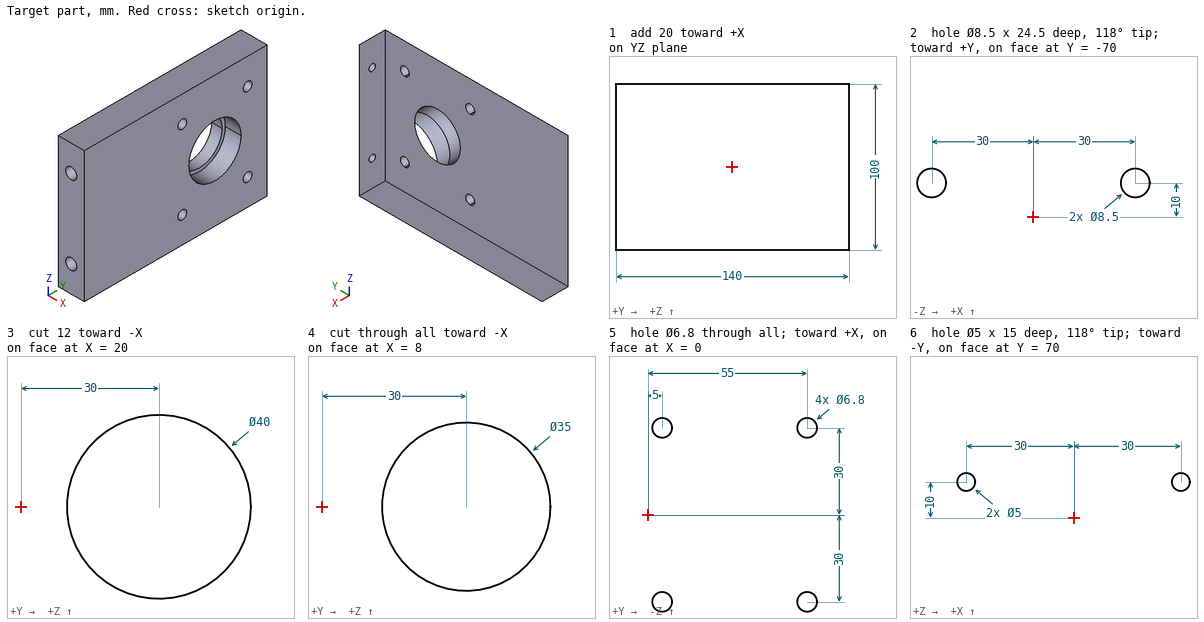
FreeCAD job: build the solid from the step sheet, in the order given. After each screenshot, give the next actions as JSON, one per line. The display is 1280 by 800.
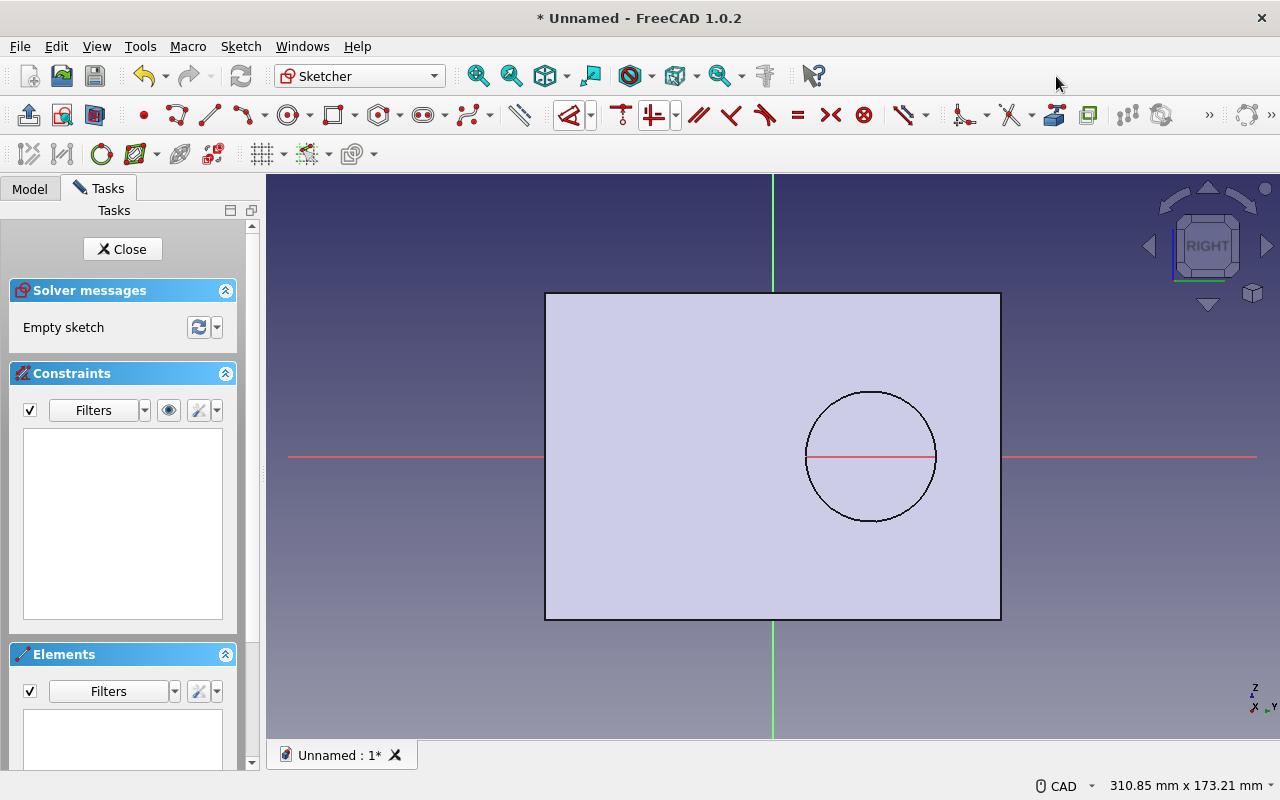
{"action": "left_click", "coordinate": [95, 116]}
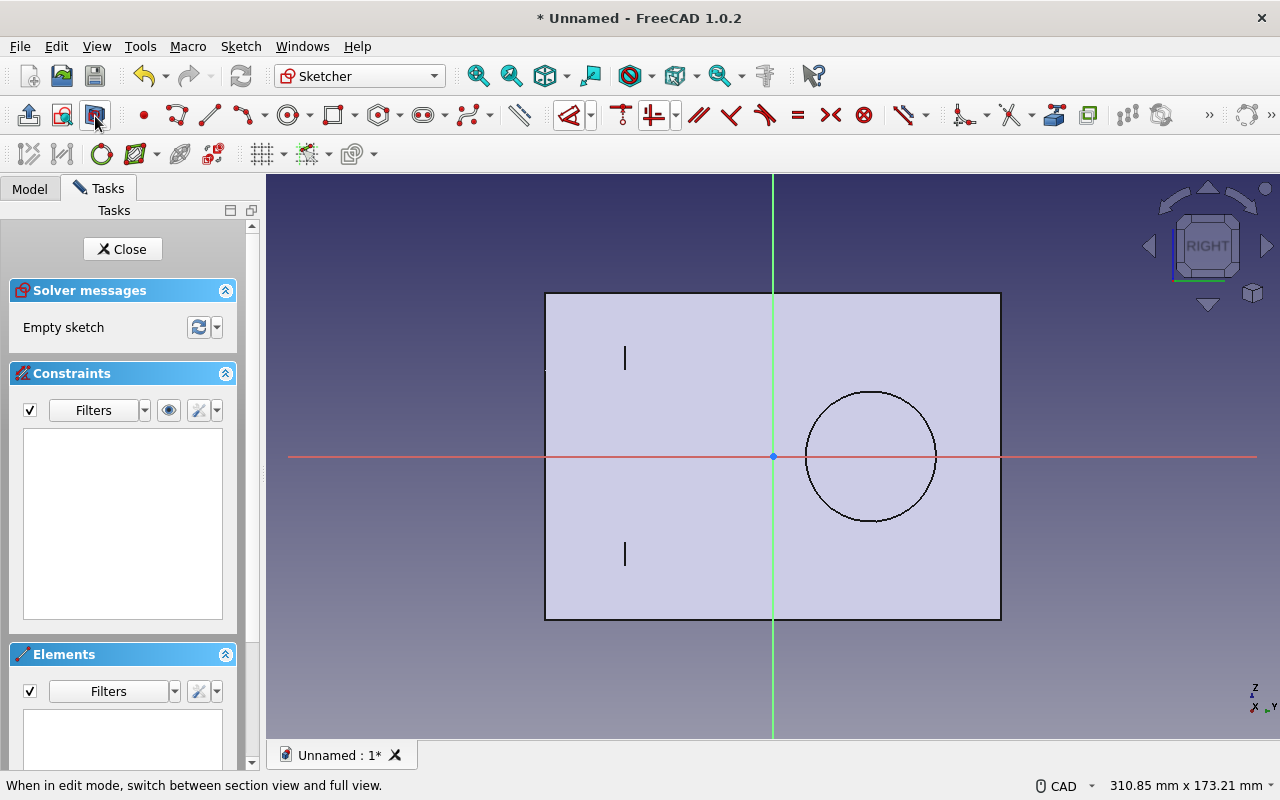
{"action": "scroll", "coordinate": [913, 456], "scroll_direction": "up", "scroll_amount": 6}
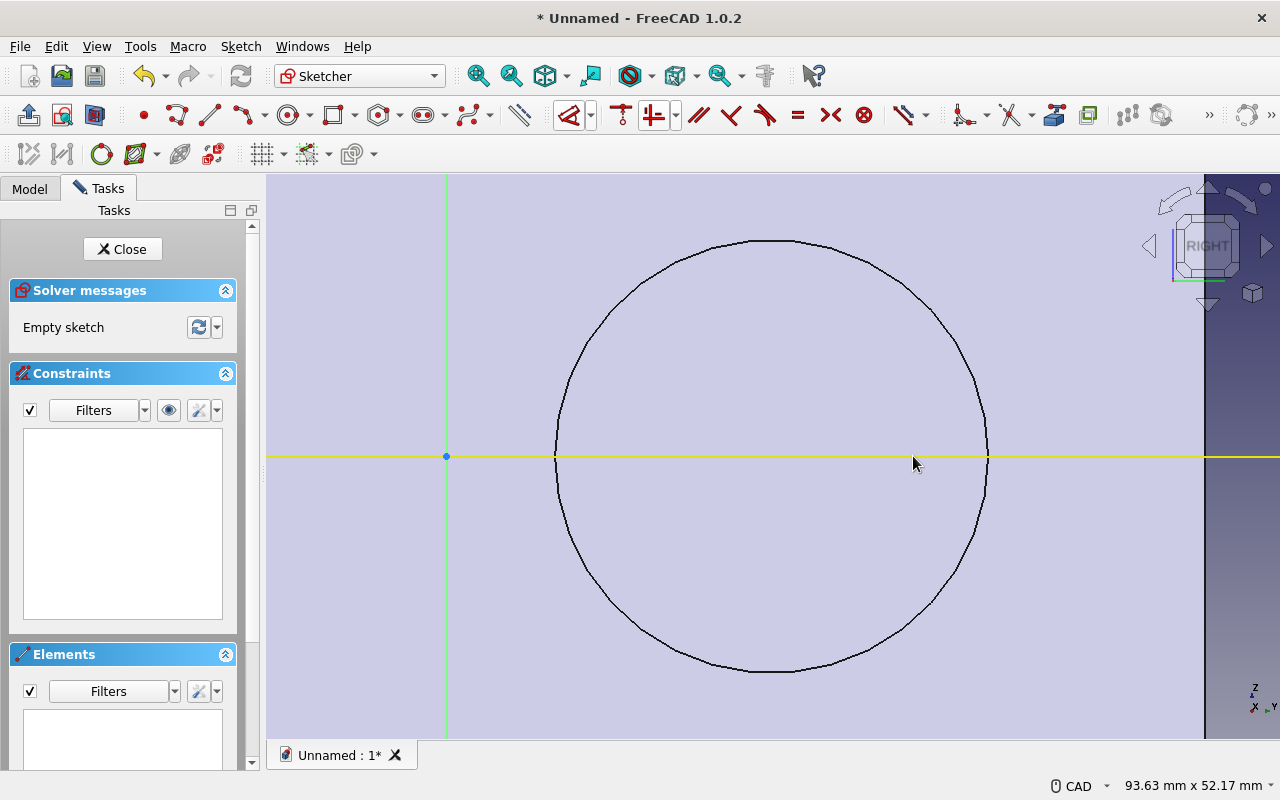
{"action": "left_click", "coordinate": [288, 116]}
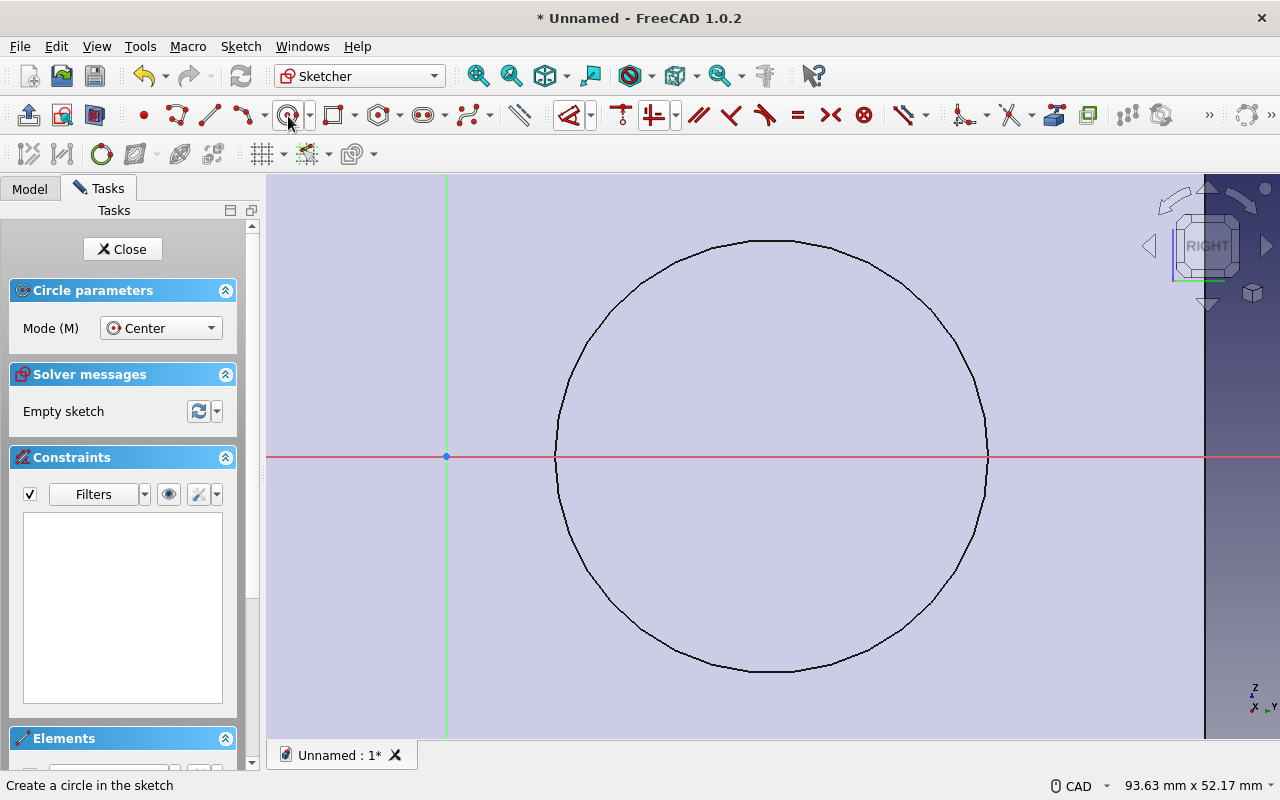
{"action": "left_click", "coordinate": [772, 456]}
{"action": "mouse_move", "coordinate": [906, 322]}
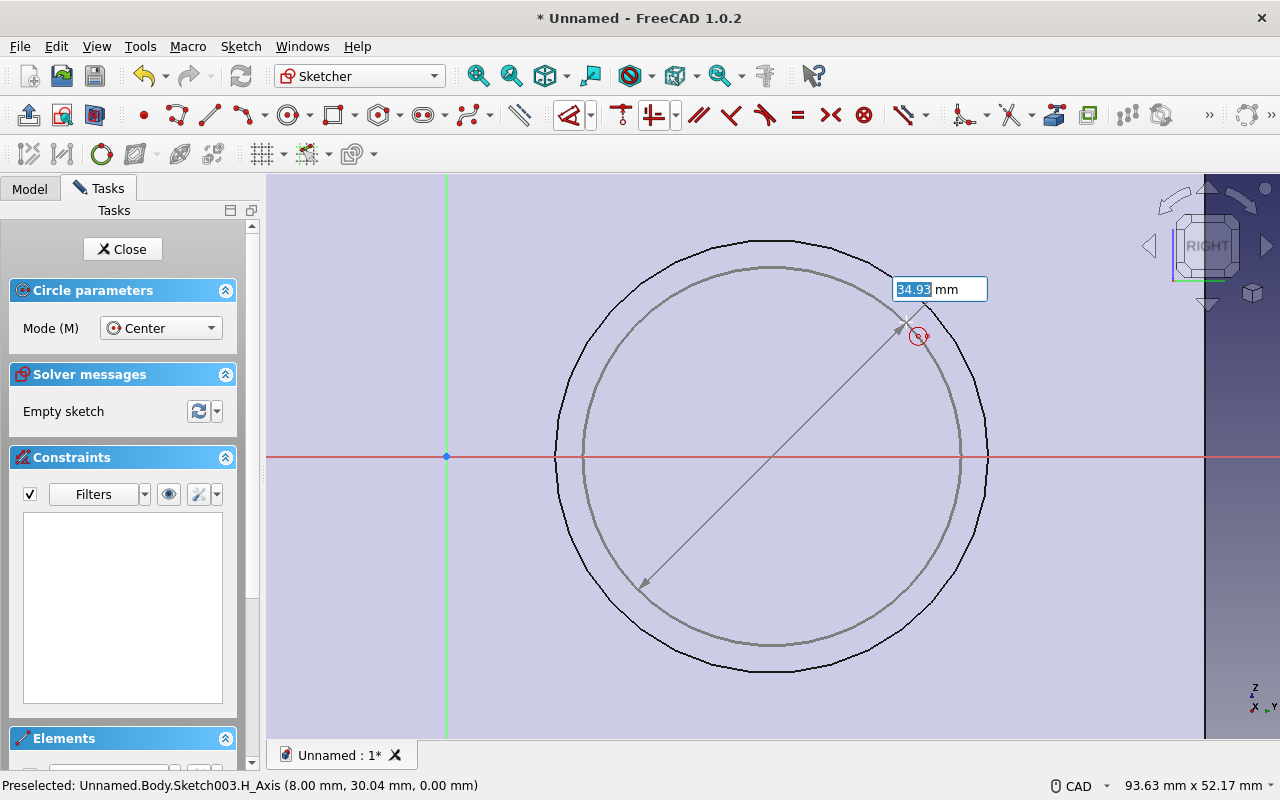
{"action": "type", "text": "35"}
{"action": "key", "text": "Return"}
{"action": "key", "text": "Escape"}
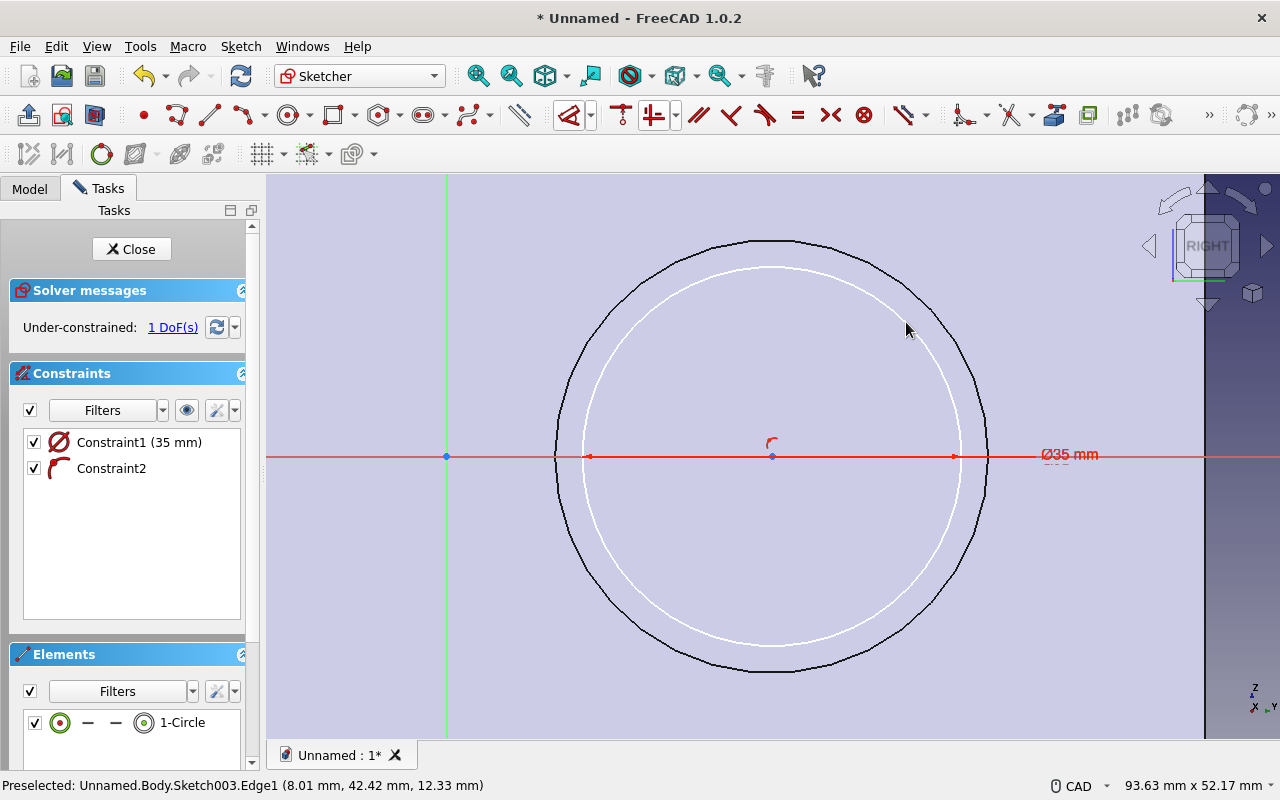
{"action": "left_click", "coordinate": [772, 456]}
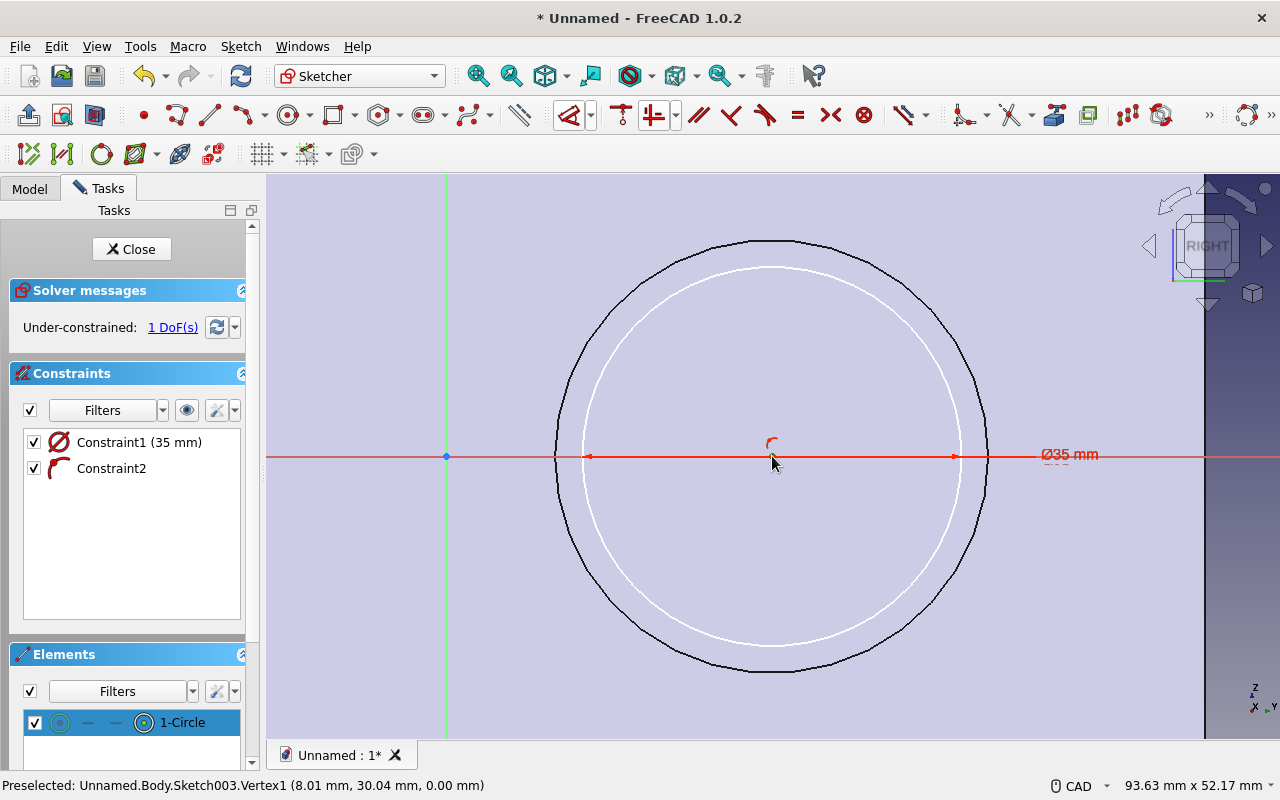
{"action": "left_click", "coordinate": [590, 116]}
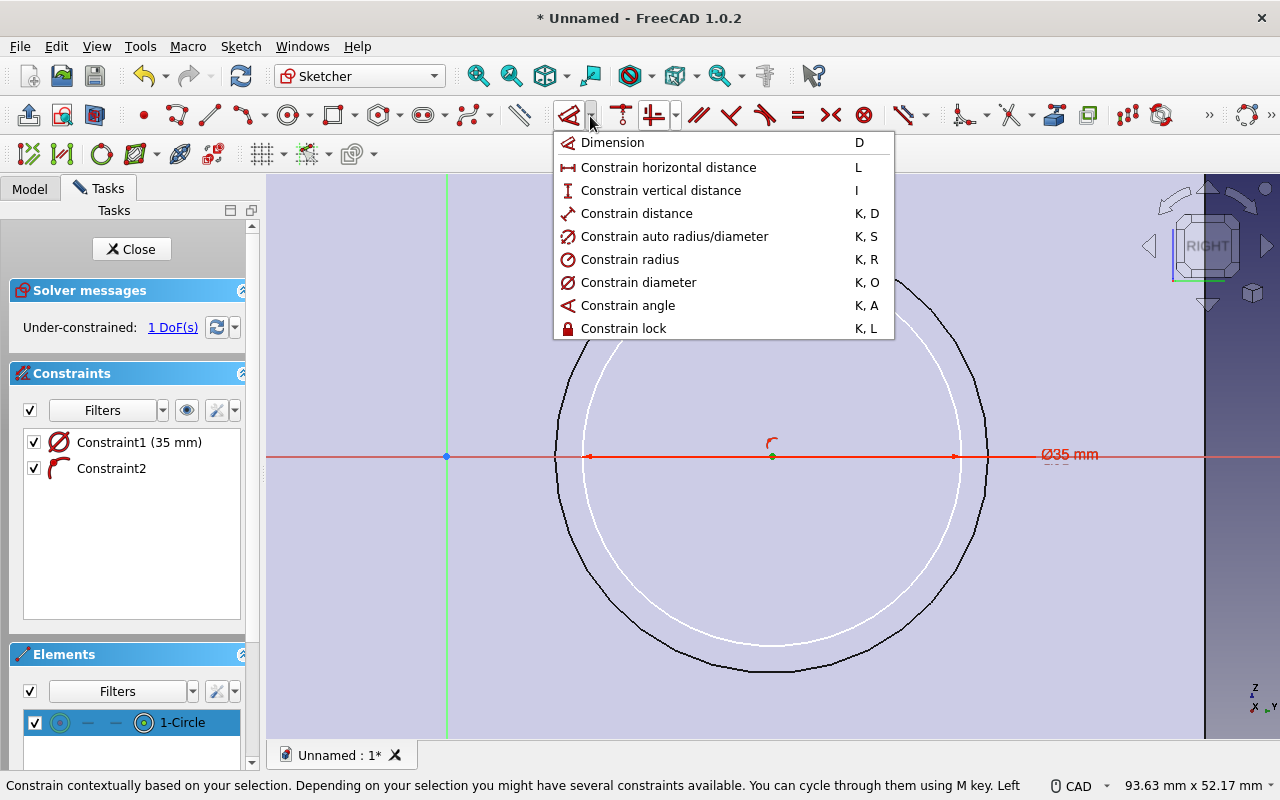
{"action": "left_click", "coordinate": [724, 168]}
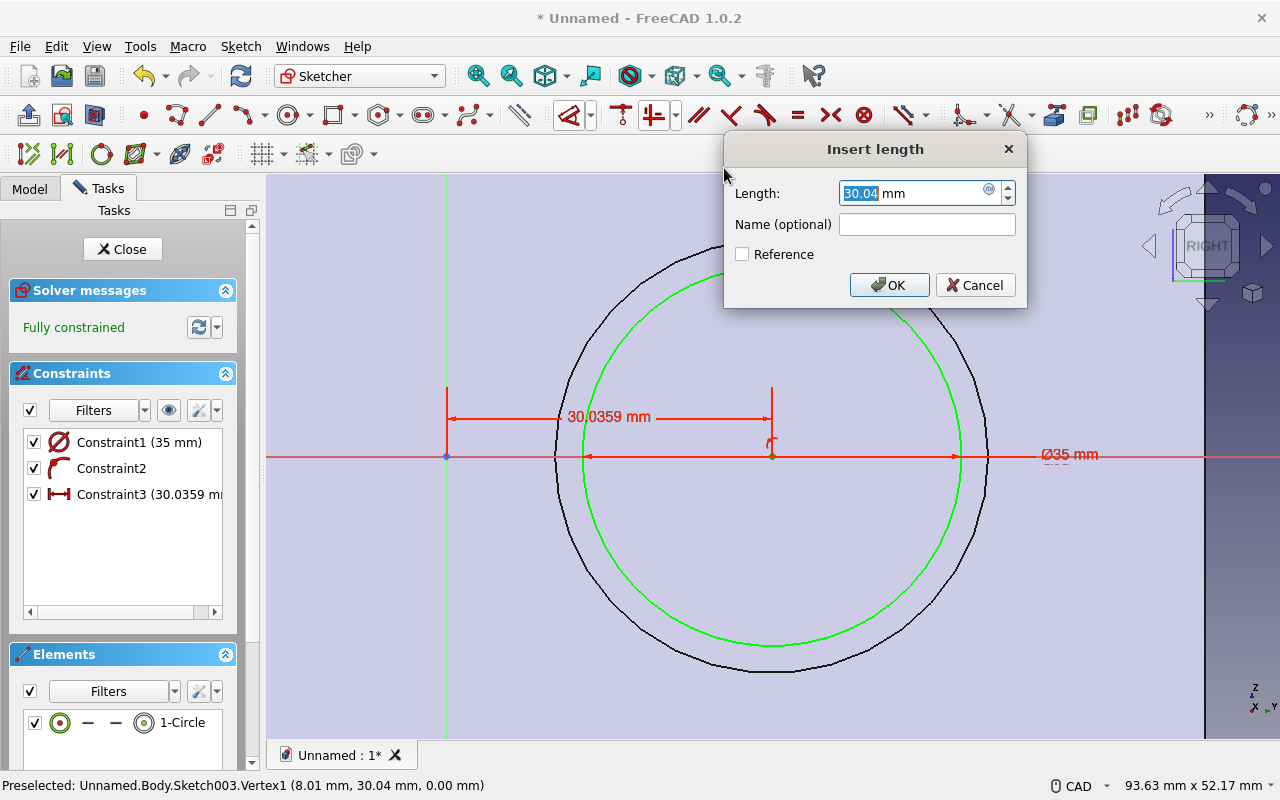
{"action": "type", "text": "30"}
{"action": "key", "text": "Return"}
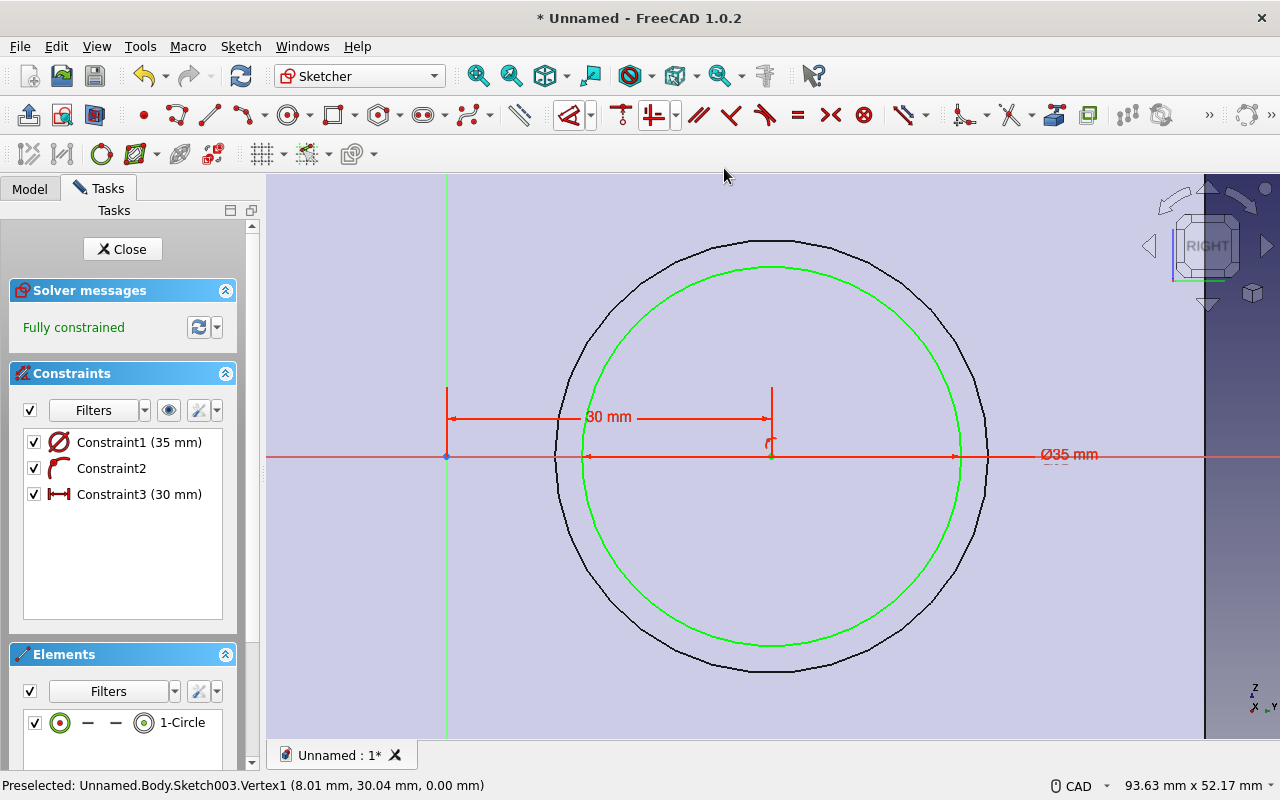
{"action": "left_click", "coordinate": [123, 249]}